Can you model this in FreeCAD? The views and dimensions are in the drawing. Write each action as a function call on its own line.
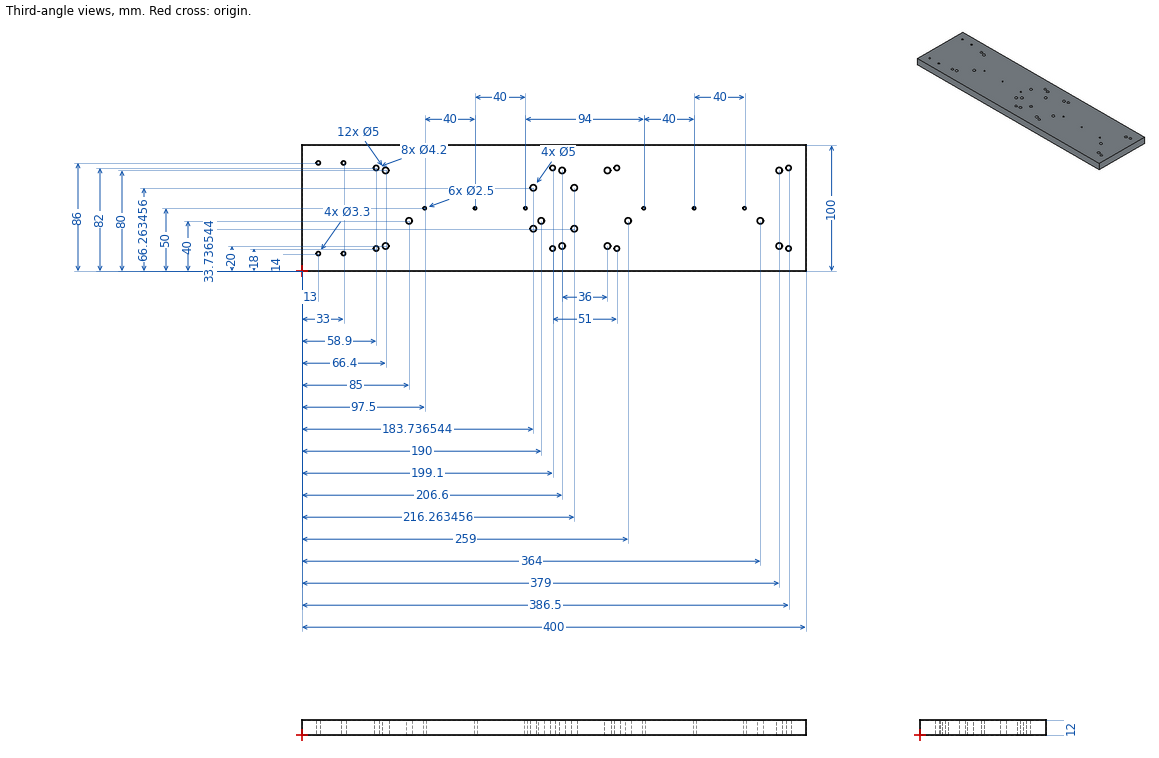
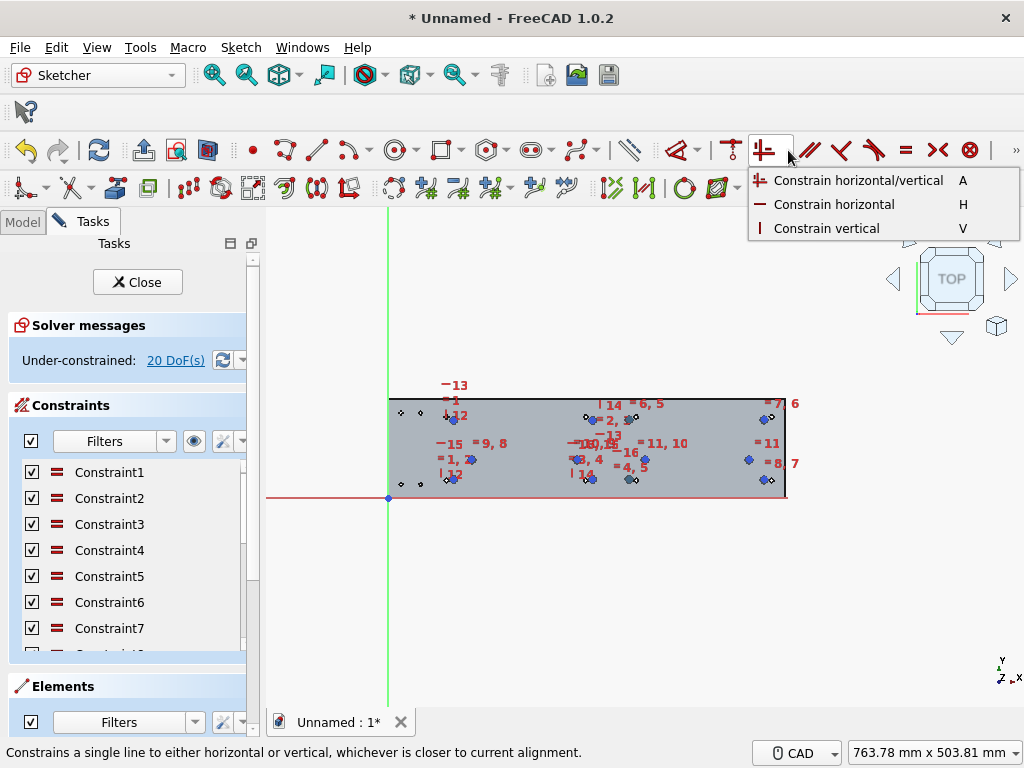
click(884, 228)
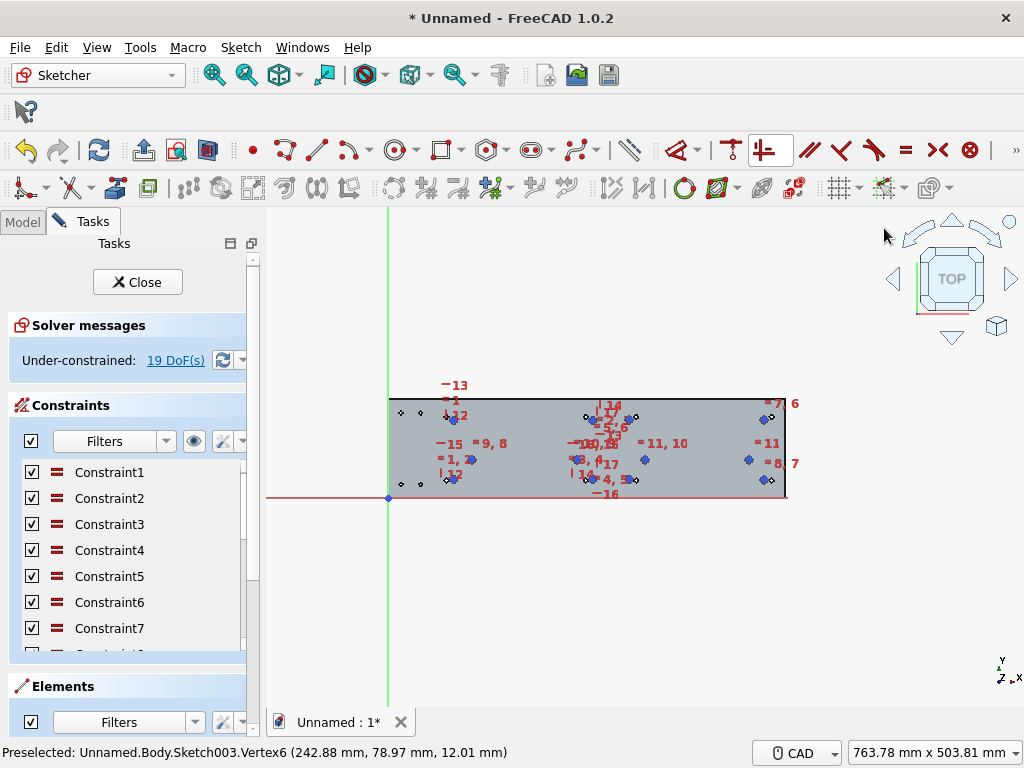
scroll(593, 420, up, 4)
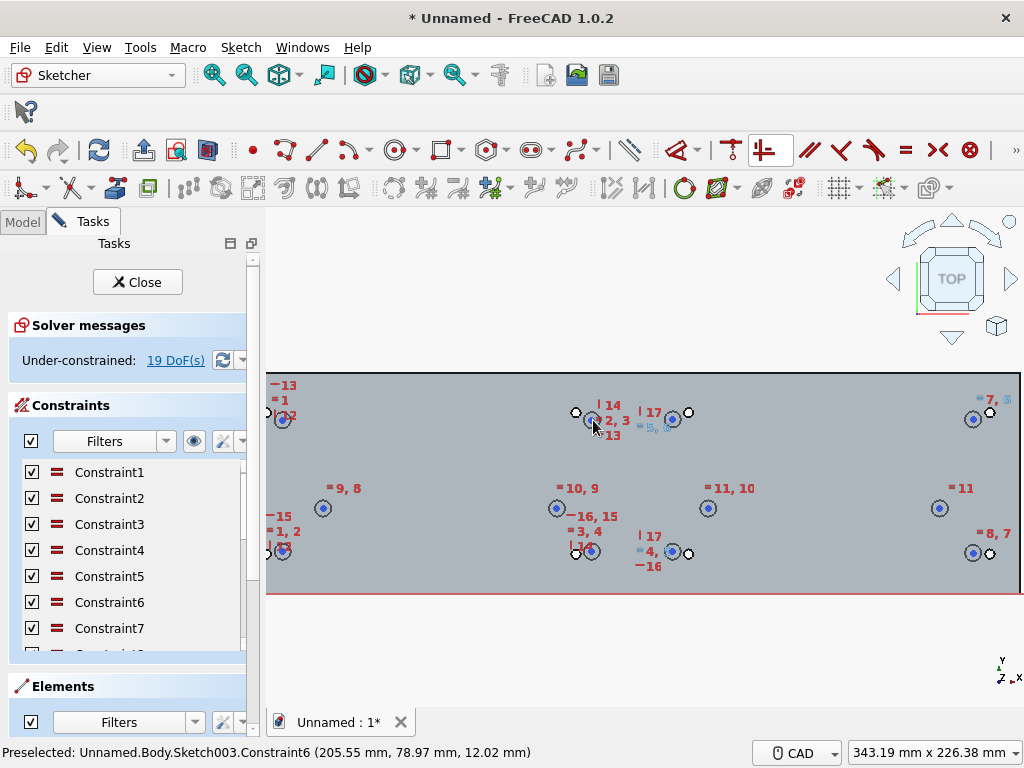
click(592, 420)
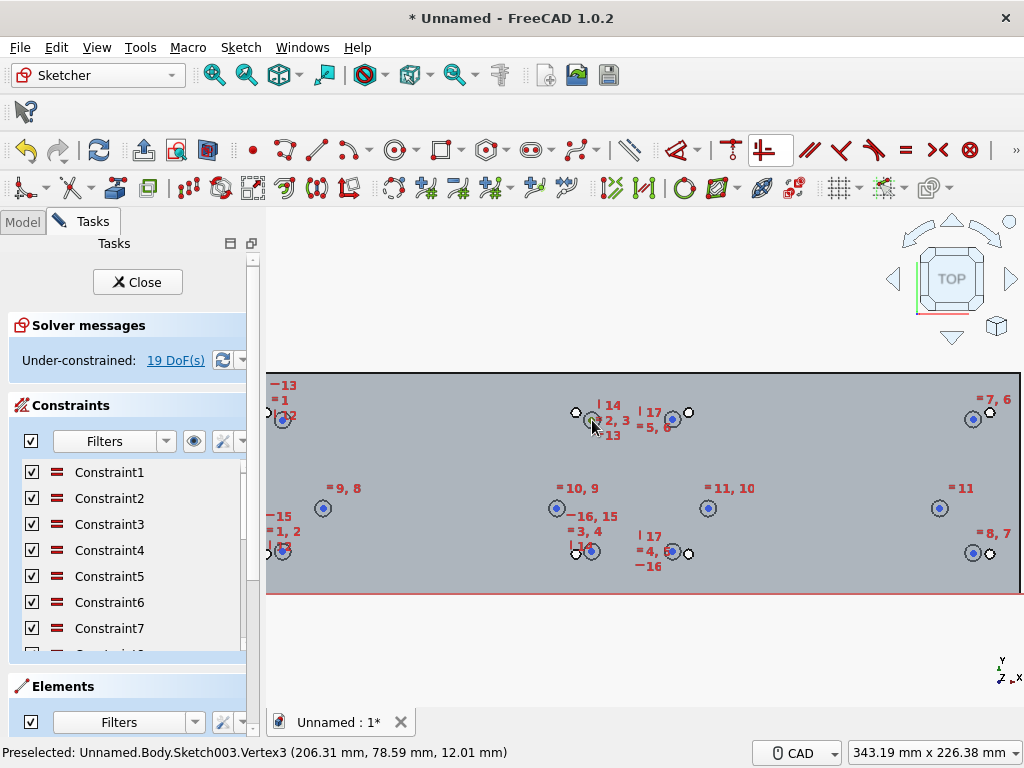
click(673, 419)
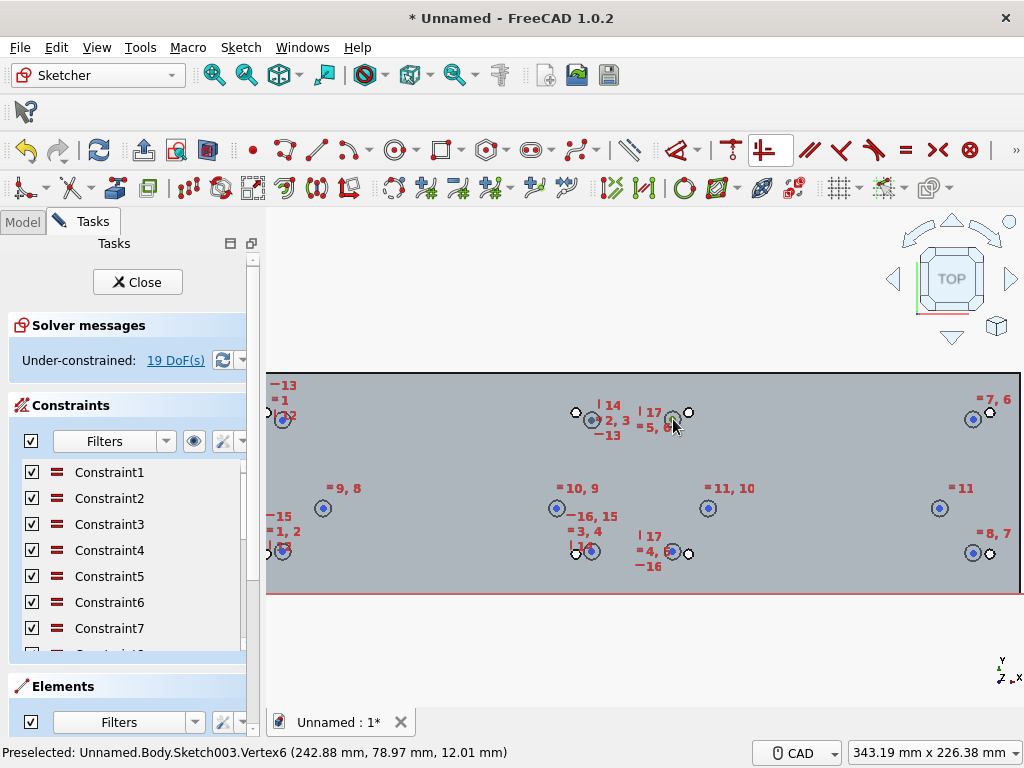
key(h)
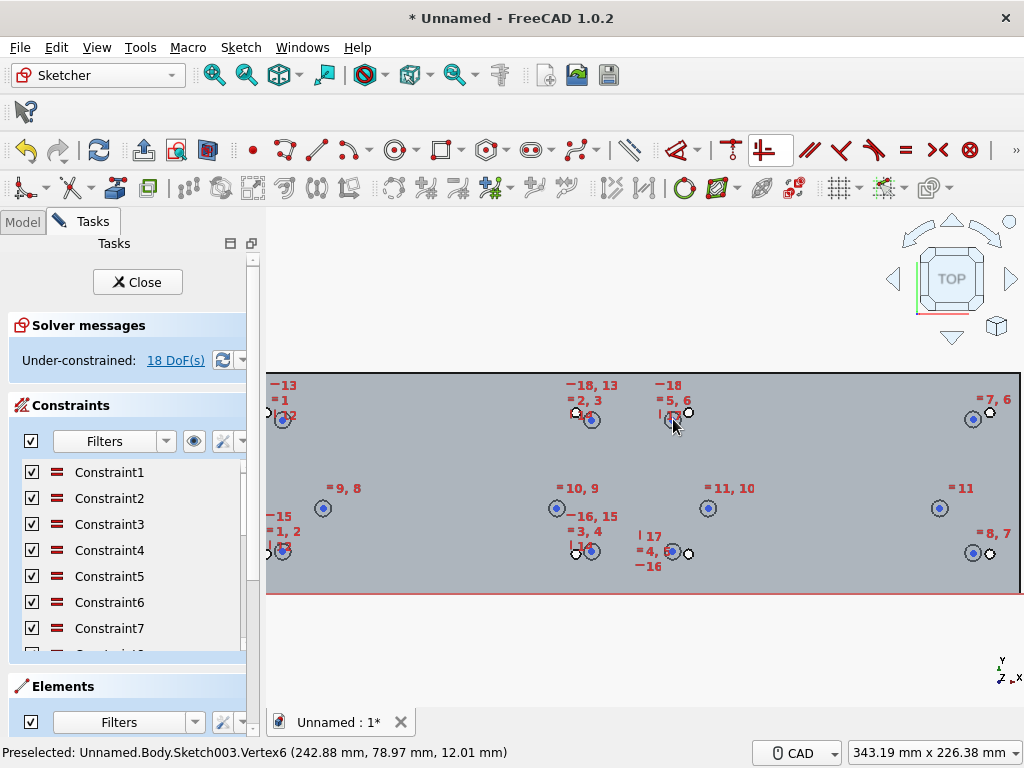
click(671, 422)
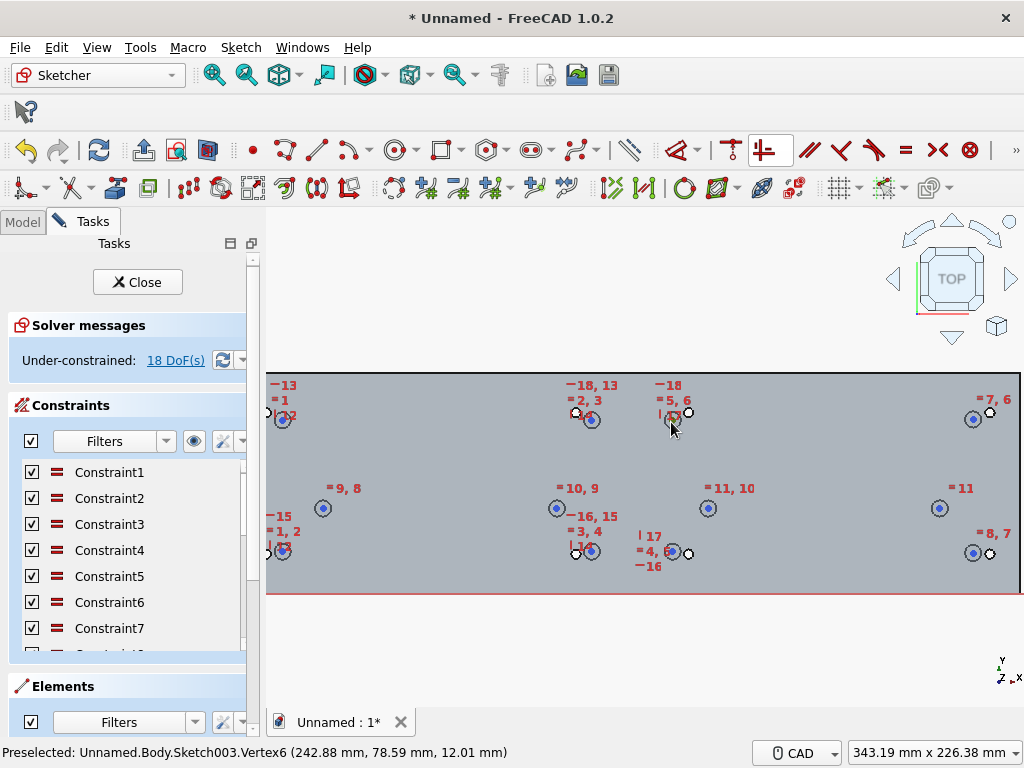
scroll(592, 420, down, 4)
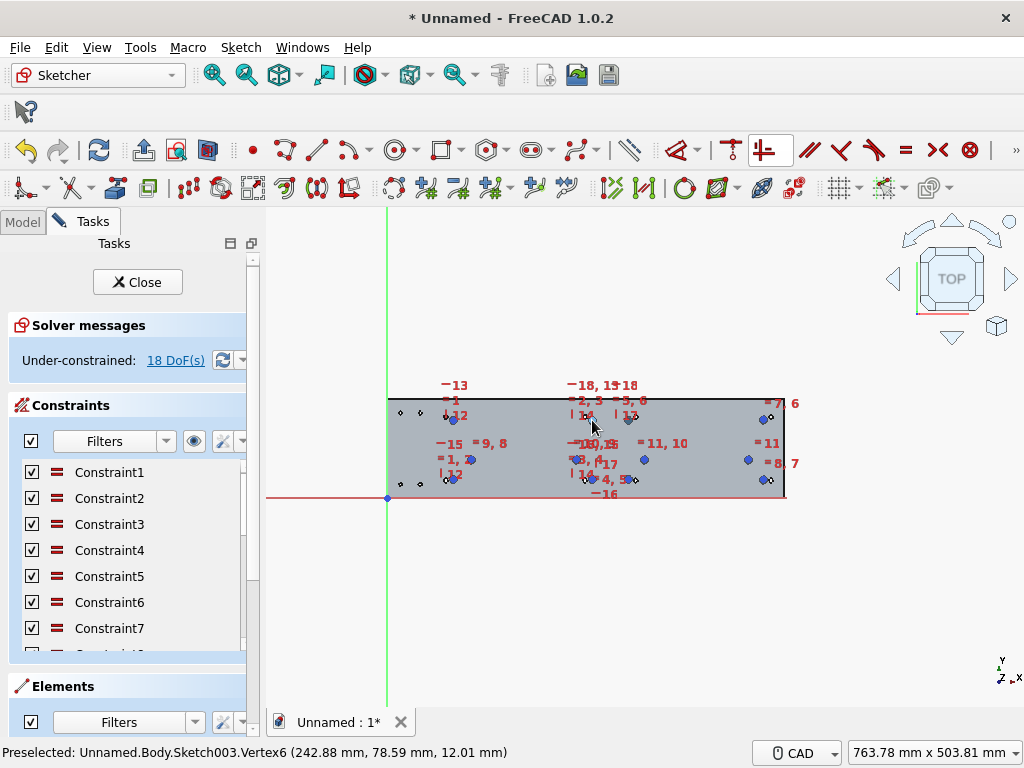
click(763, 420)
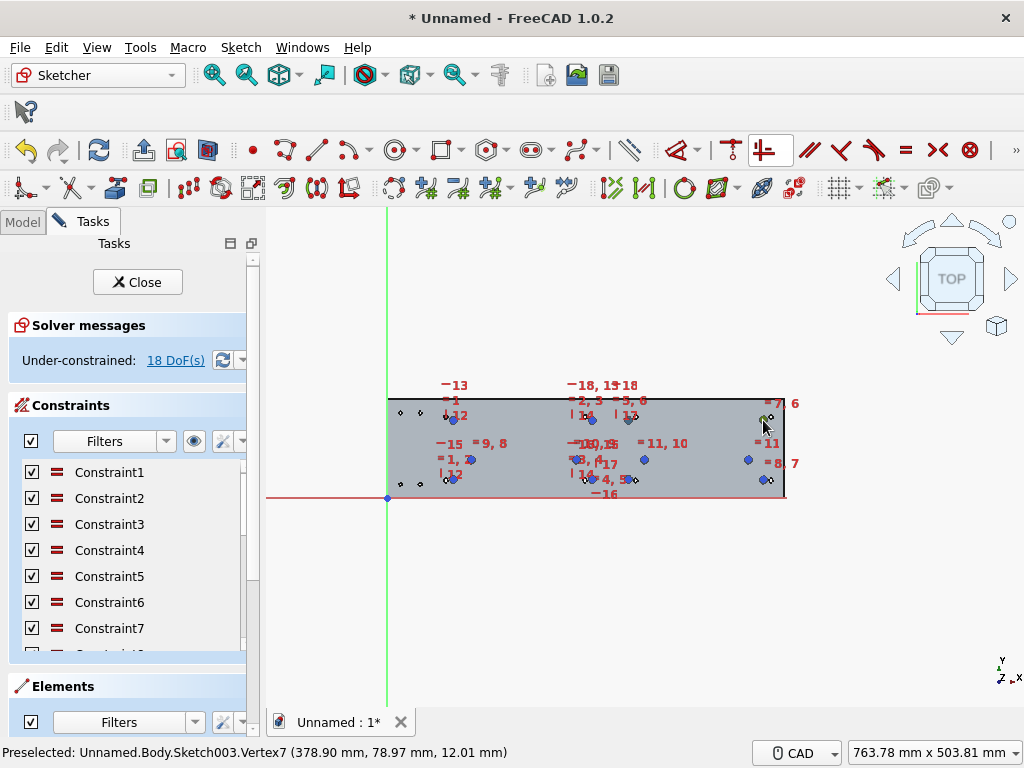
click(788, 150)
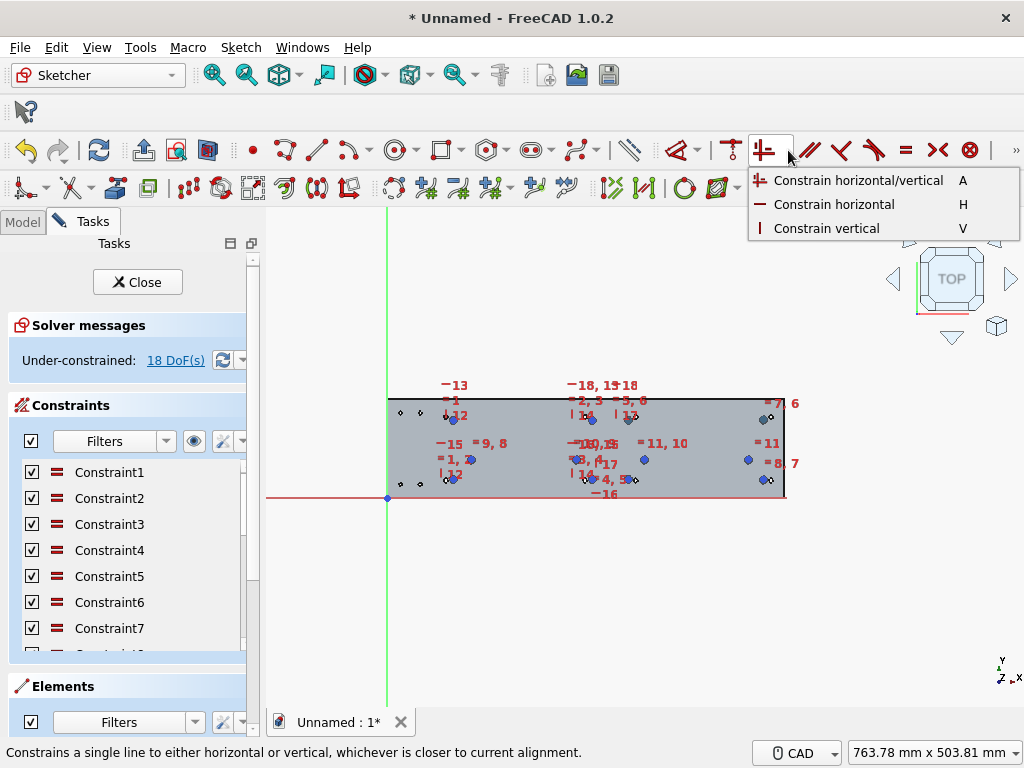
click(884, 204)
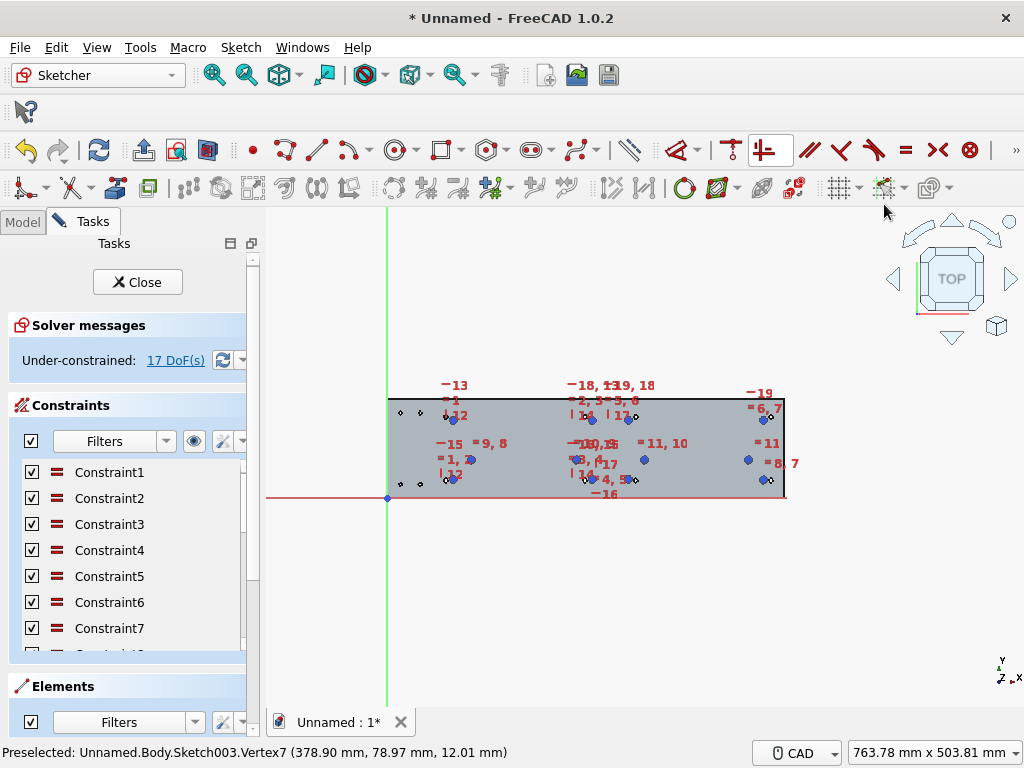
click(763, 420)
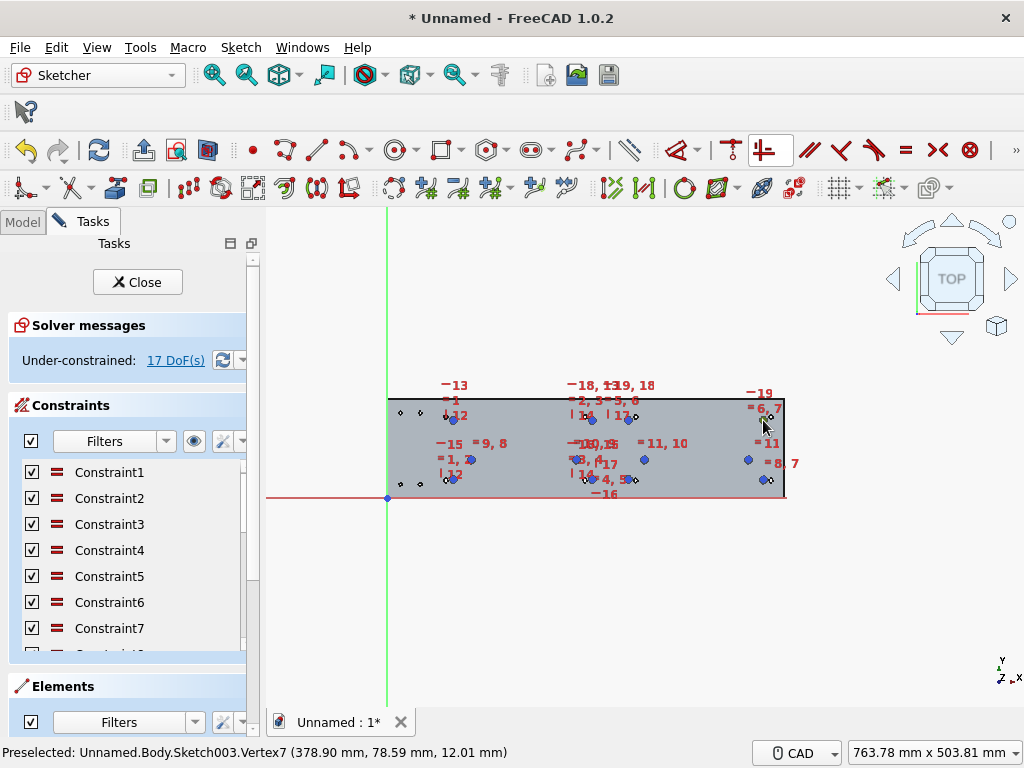
click(763, 480)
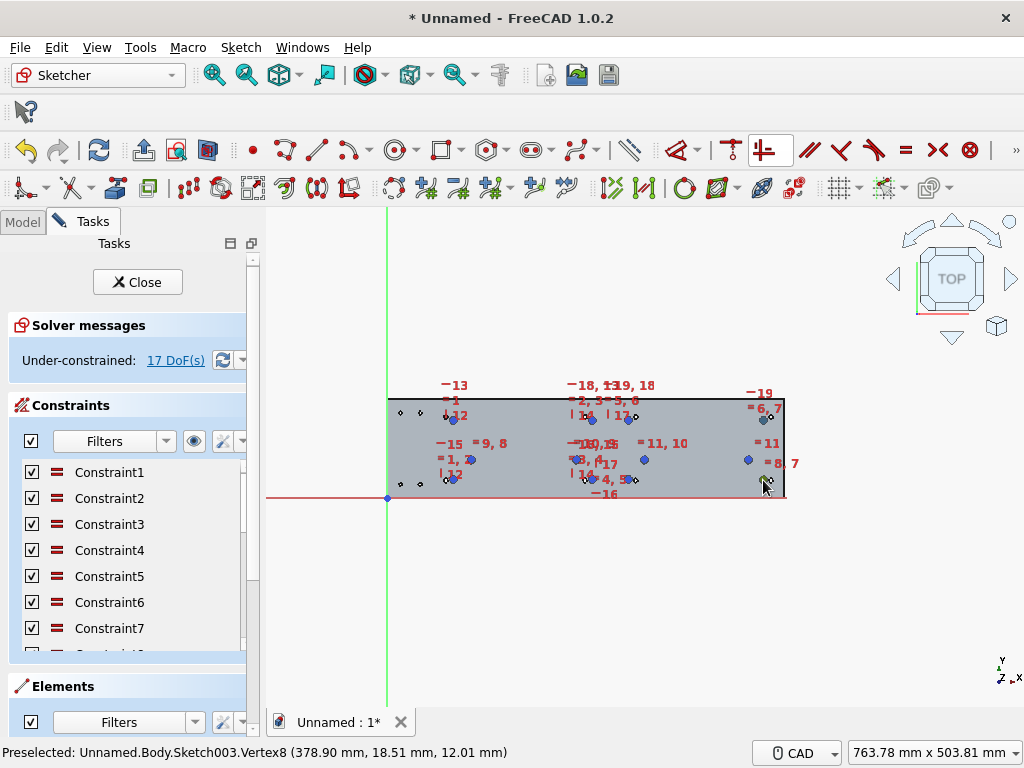
key(v)